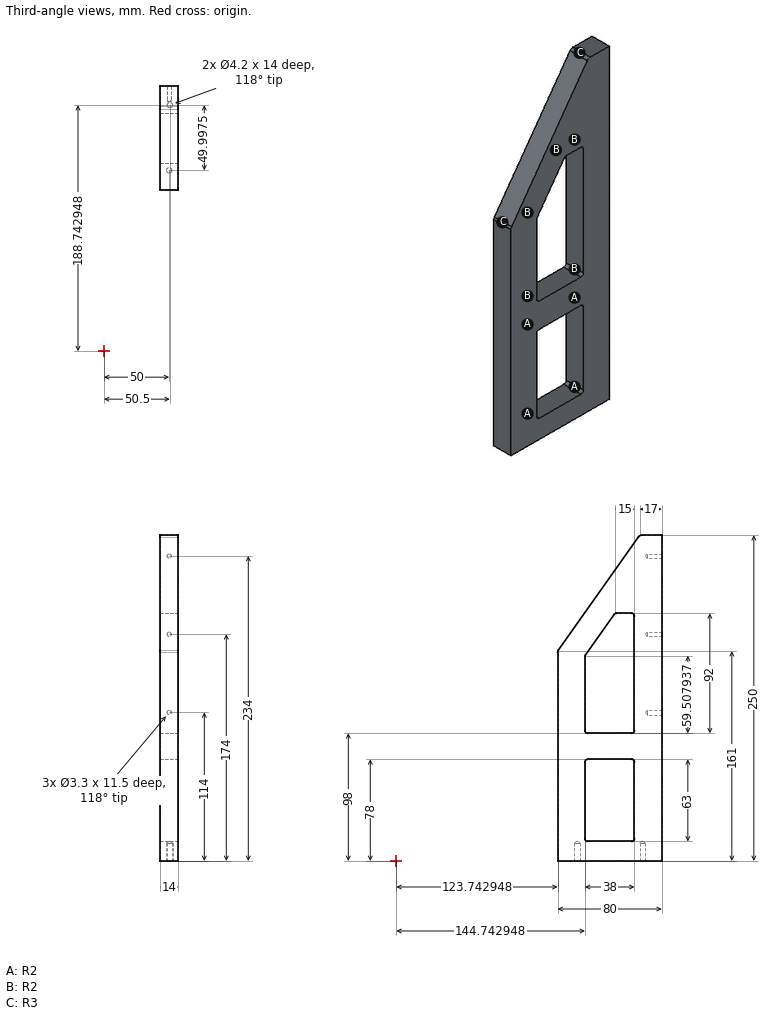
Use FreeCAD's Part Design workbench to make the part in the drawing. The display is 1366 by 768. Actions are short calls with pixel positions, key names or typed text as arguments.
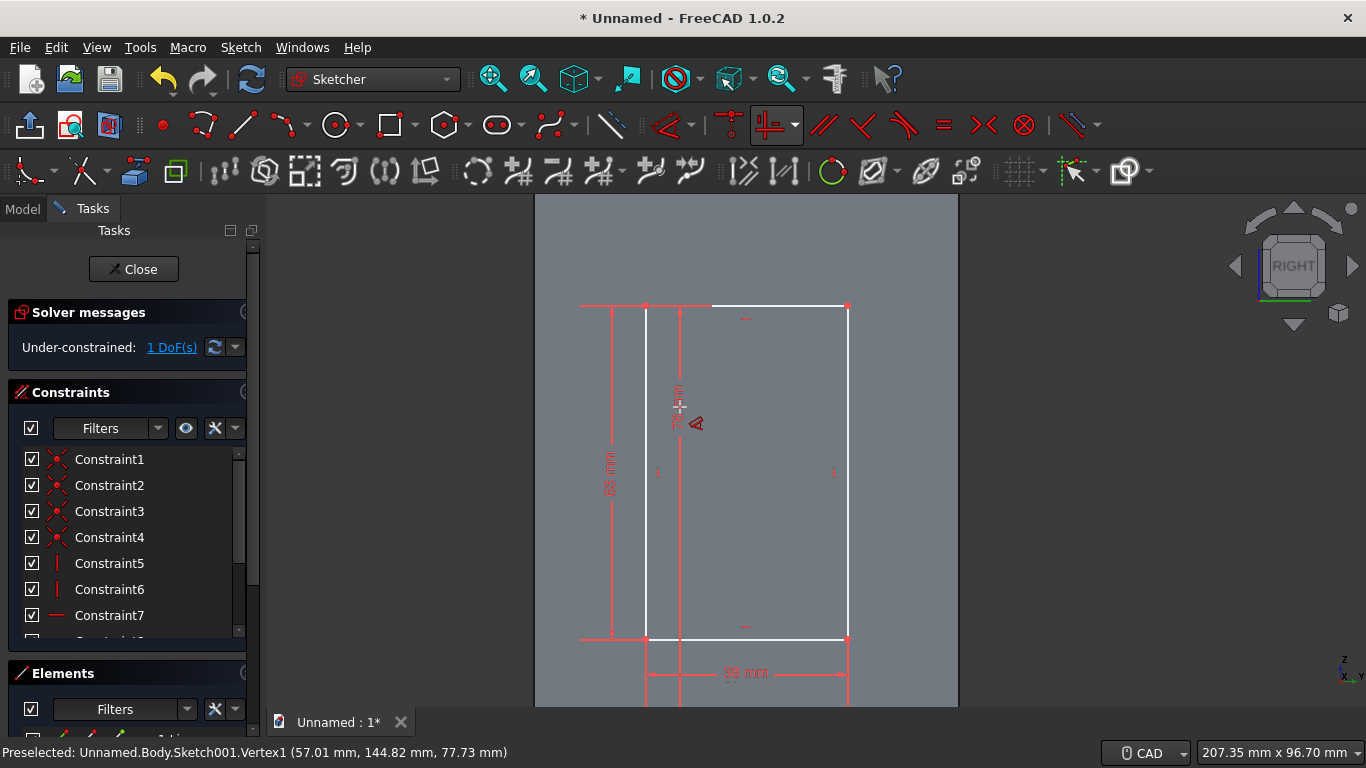
click(646, 306)
click(470, 272)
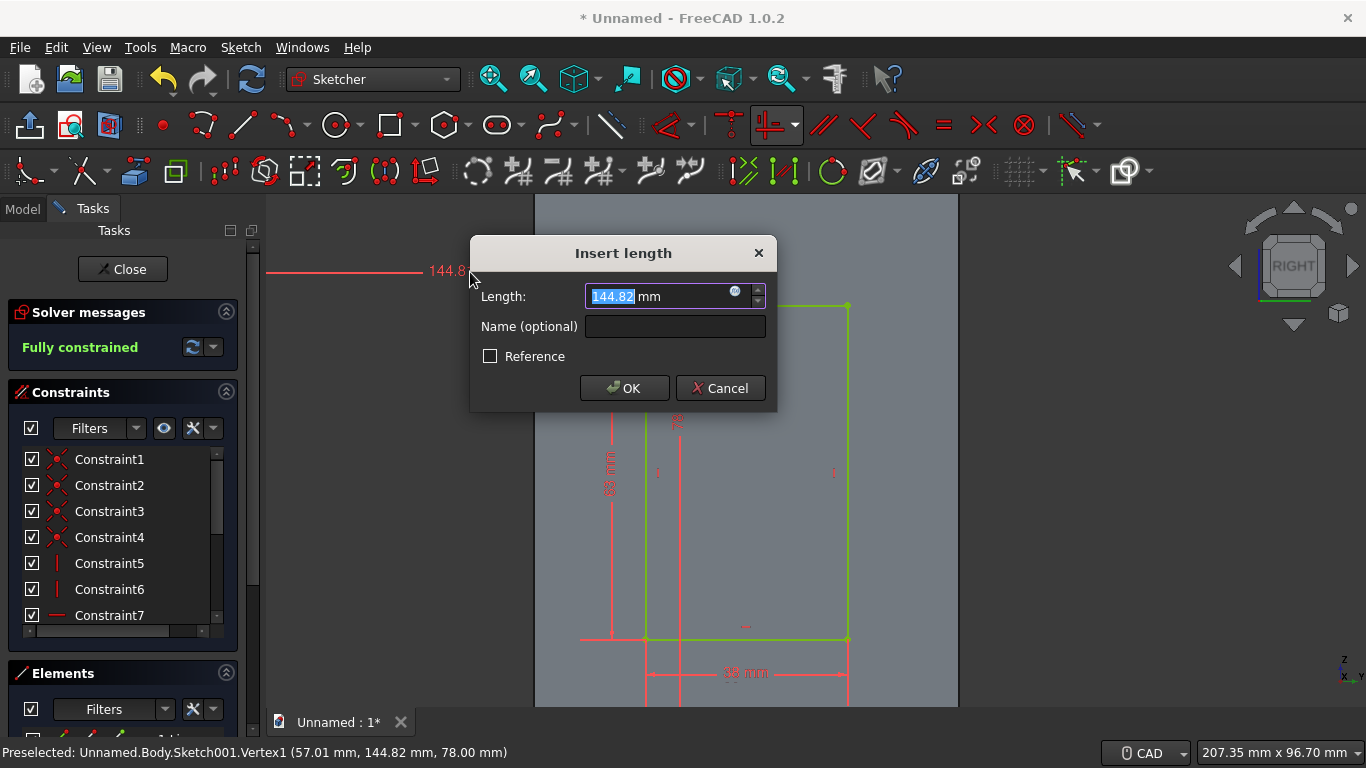
text(144.742948)
key(Return)
key(Escape)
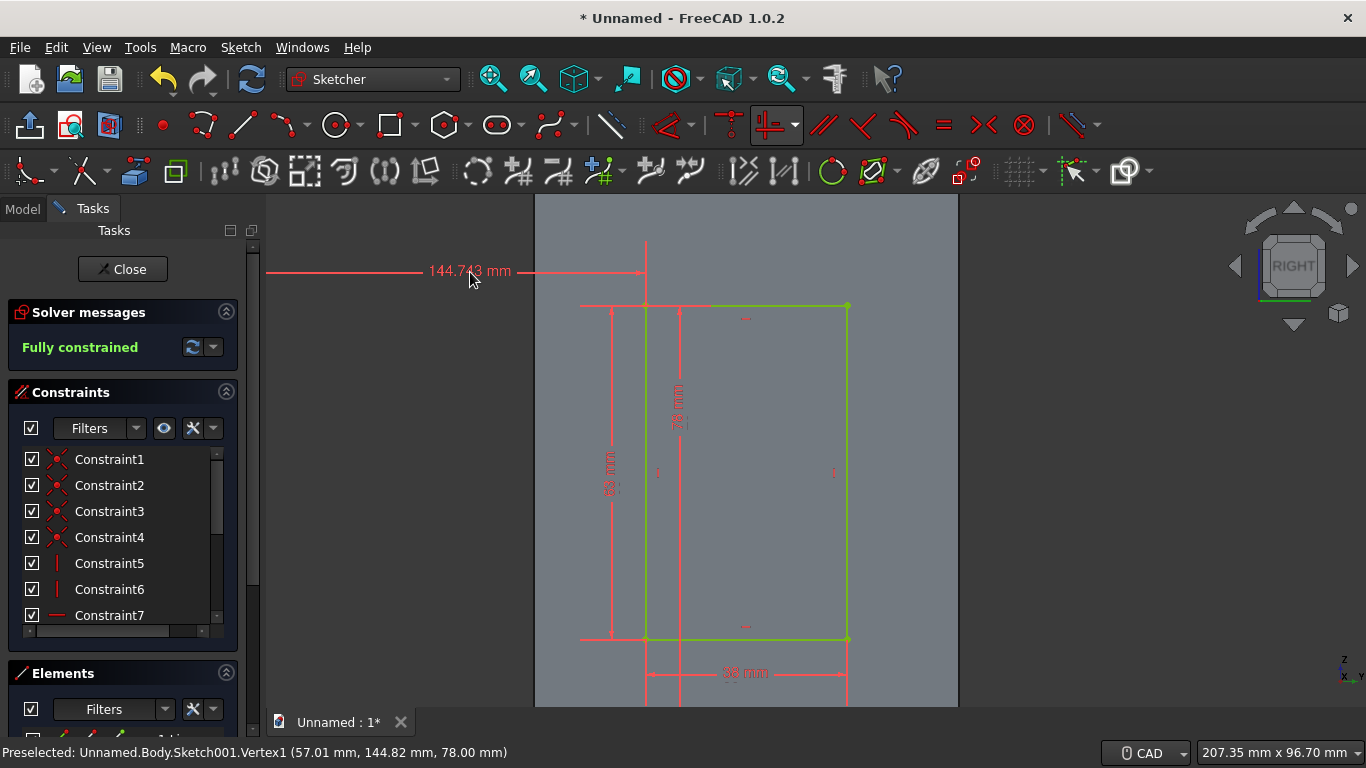
click(123, 269)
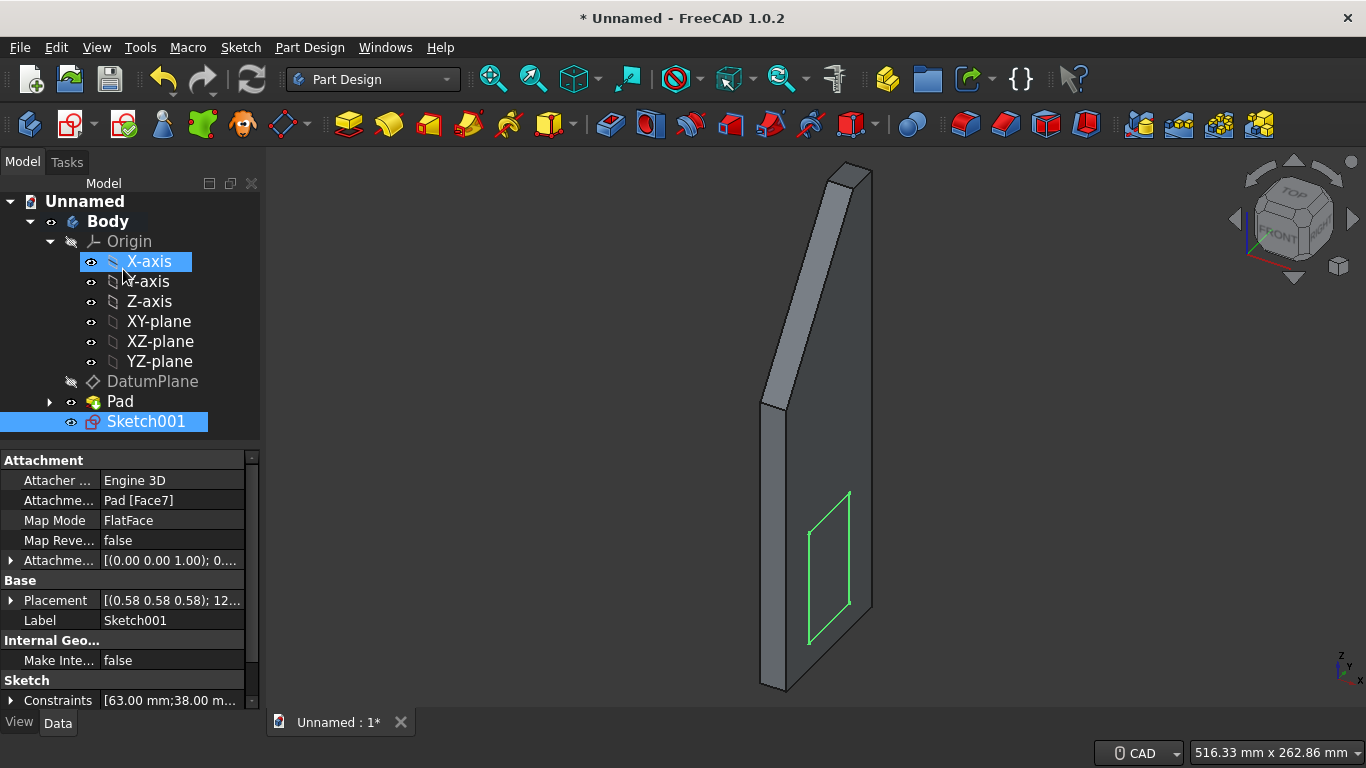
click(612, 124)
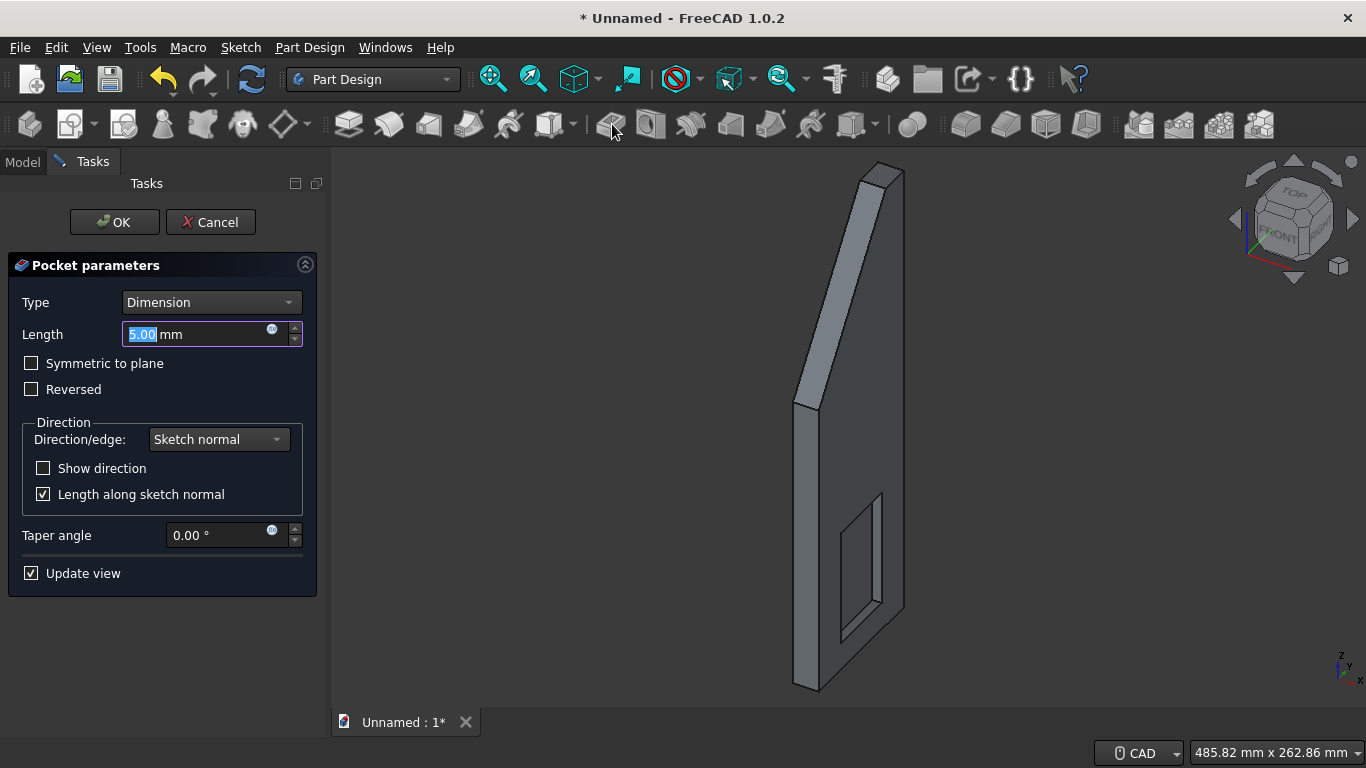
click(212, 302)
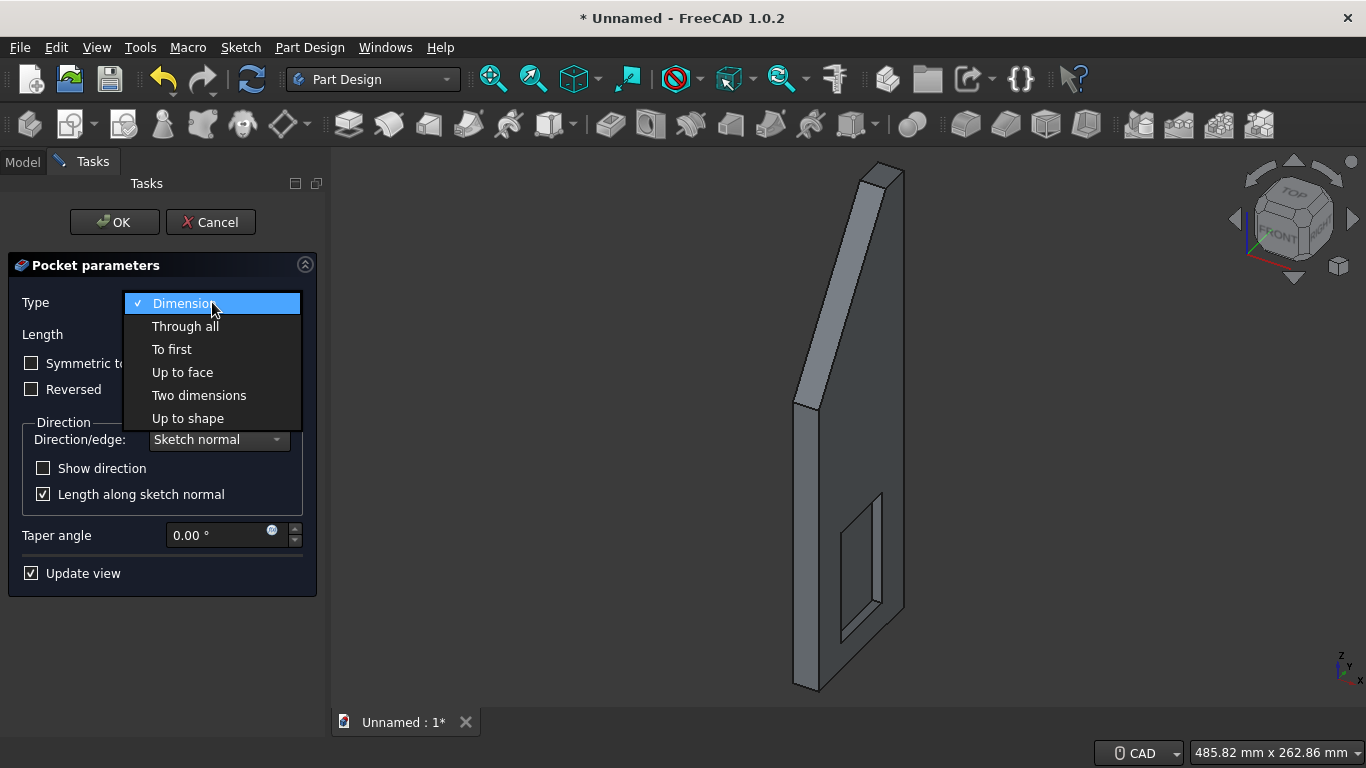
click(212, 326)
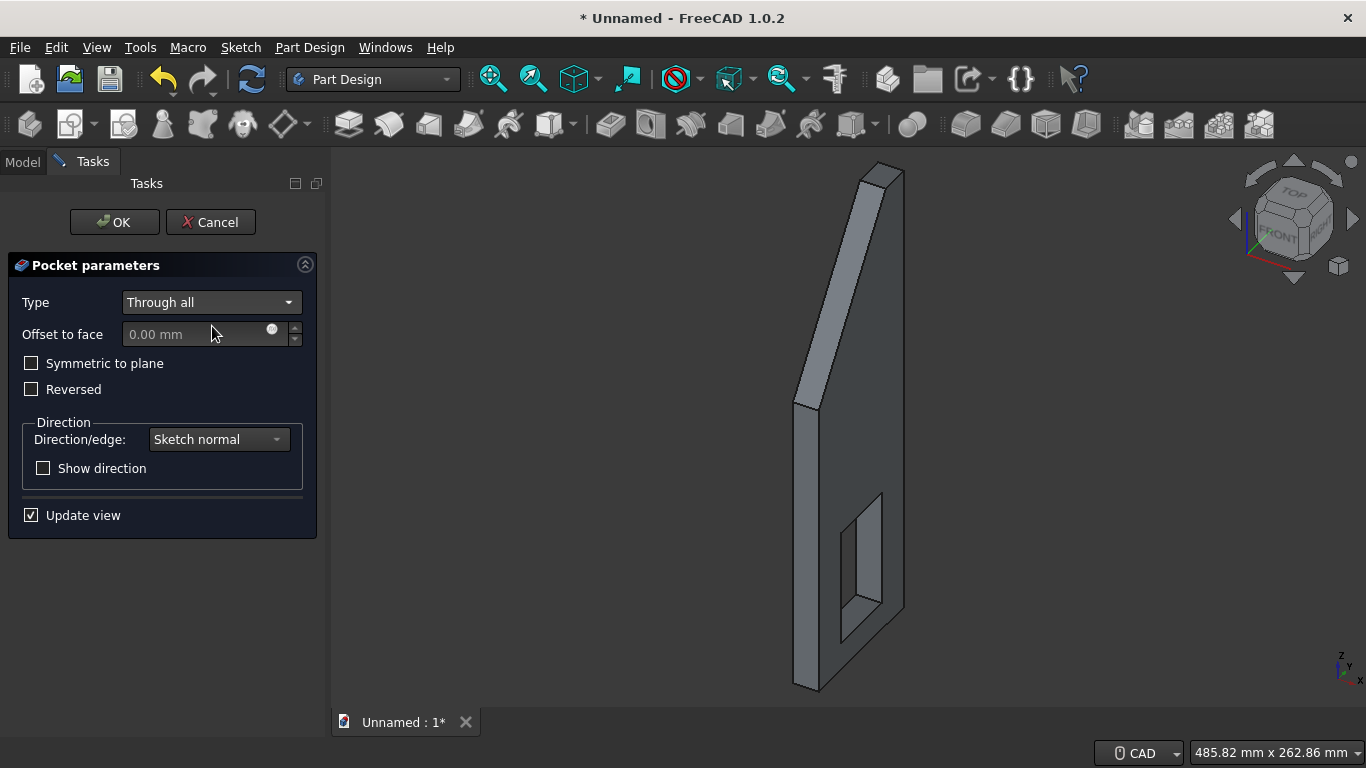
click(115, 222)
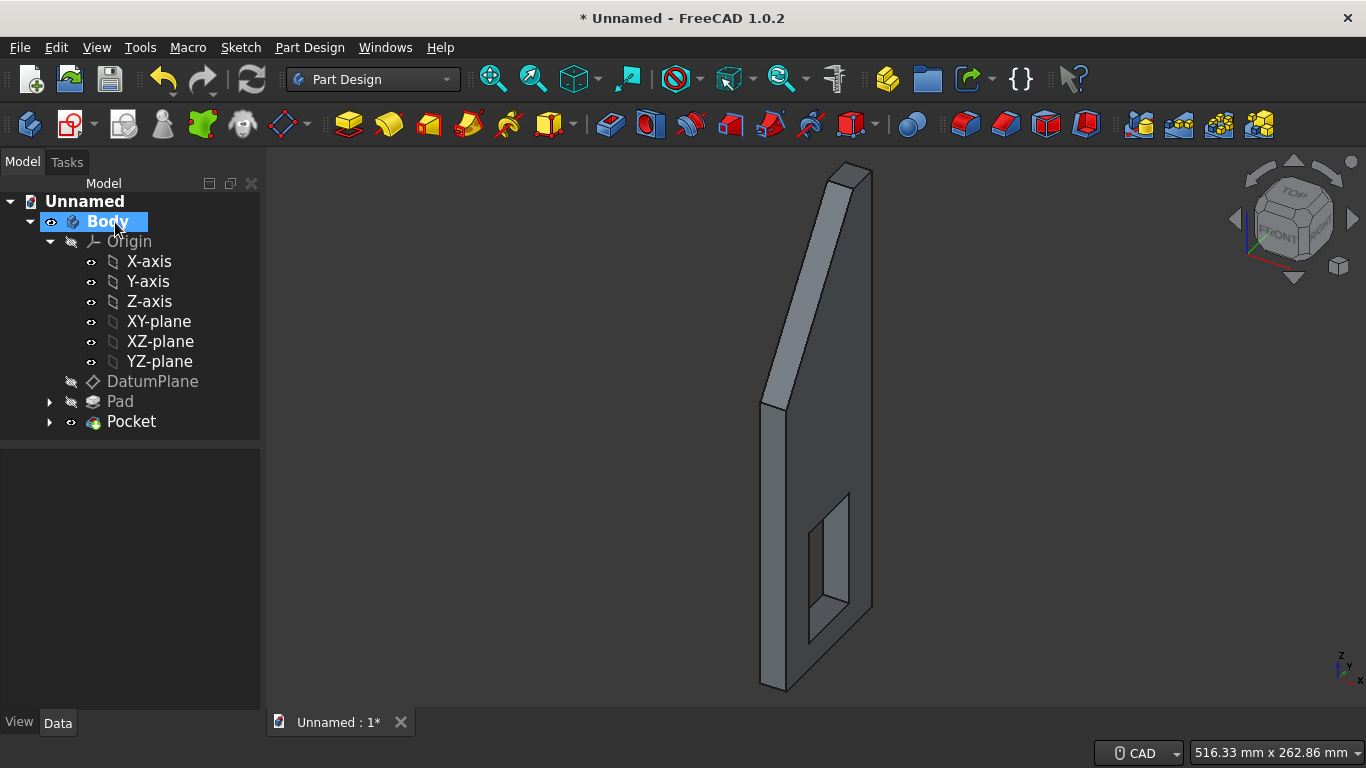
key(0)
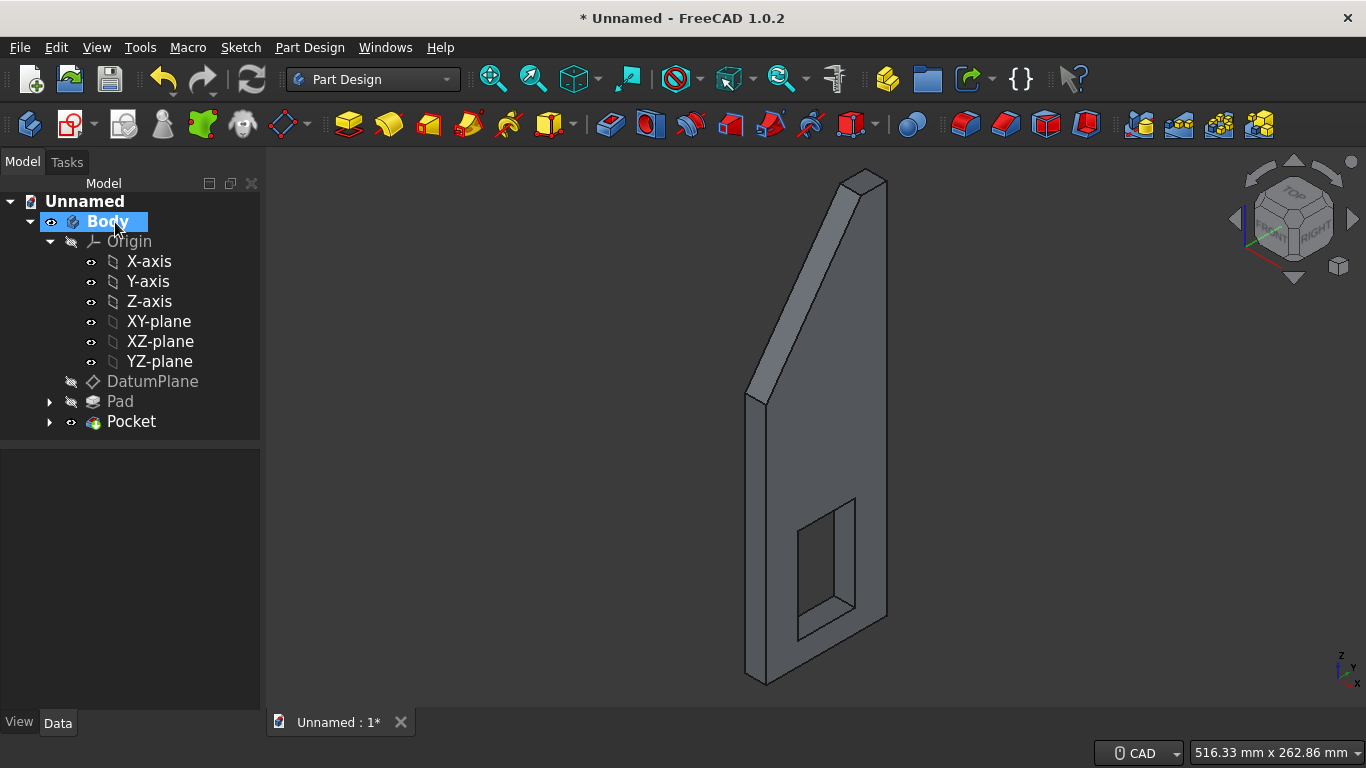
key(2)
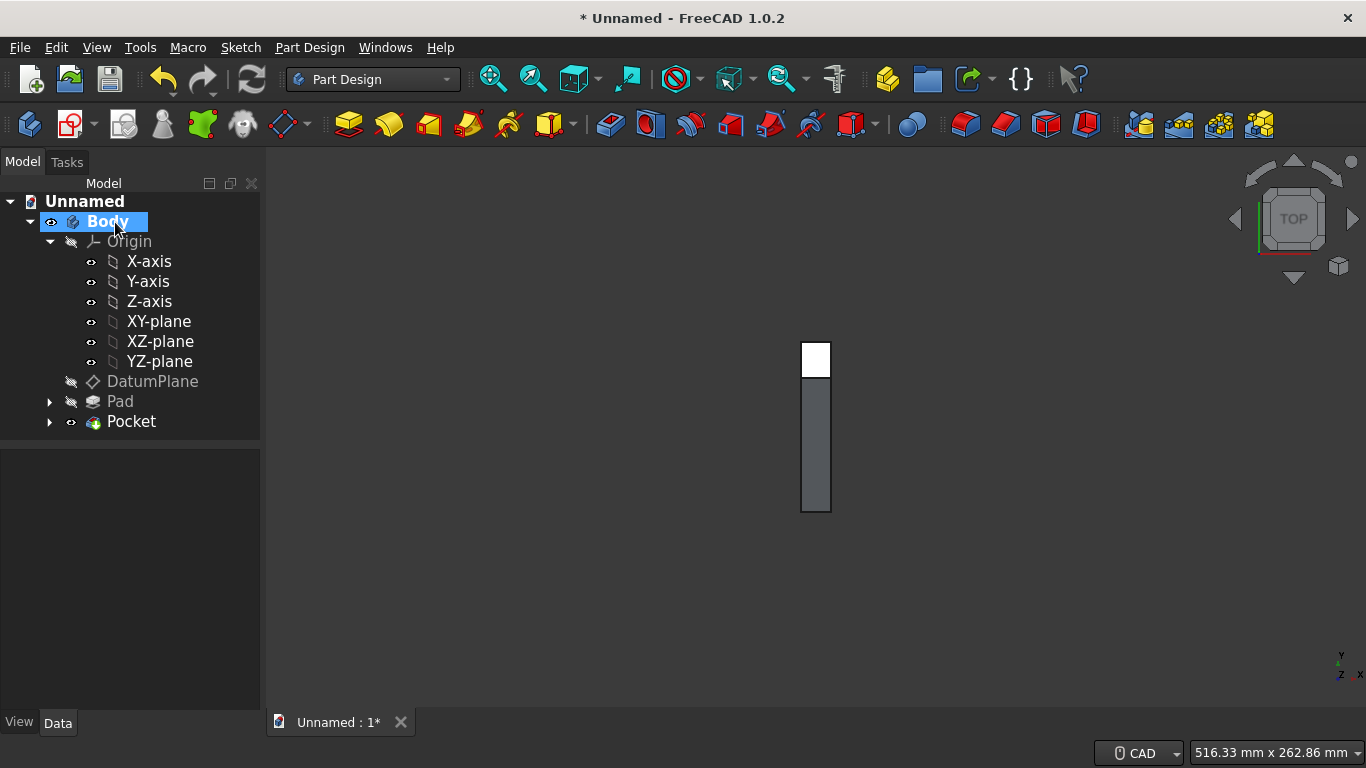
click(494, 80)